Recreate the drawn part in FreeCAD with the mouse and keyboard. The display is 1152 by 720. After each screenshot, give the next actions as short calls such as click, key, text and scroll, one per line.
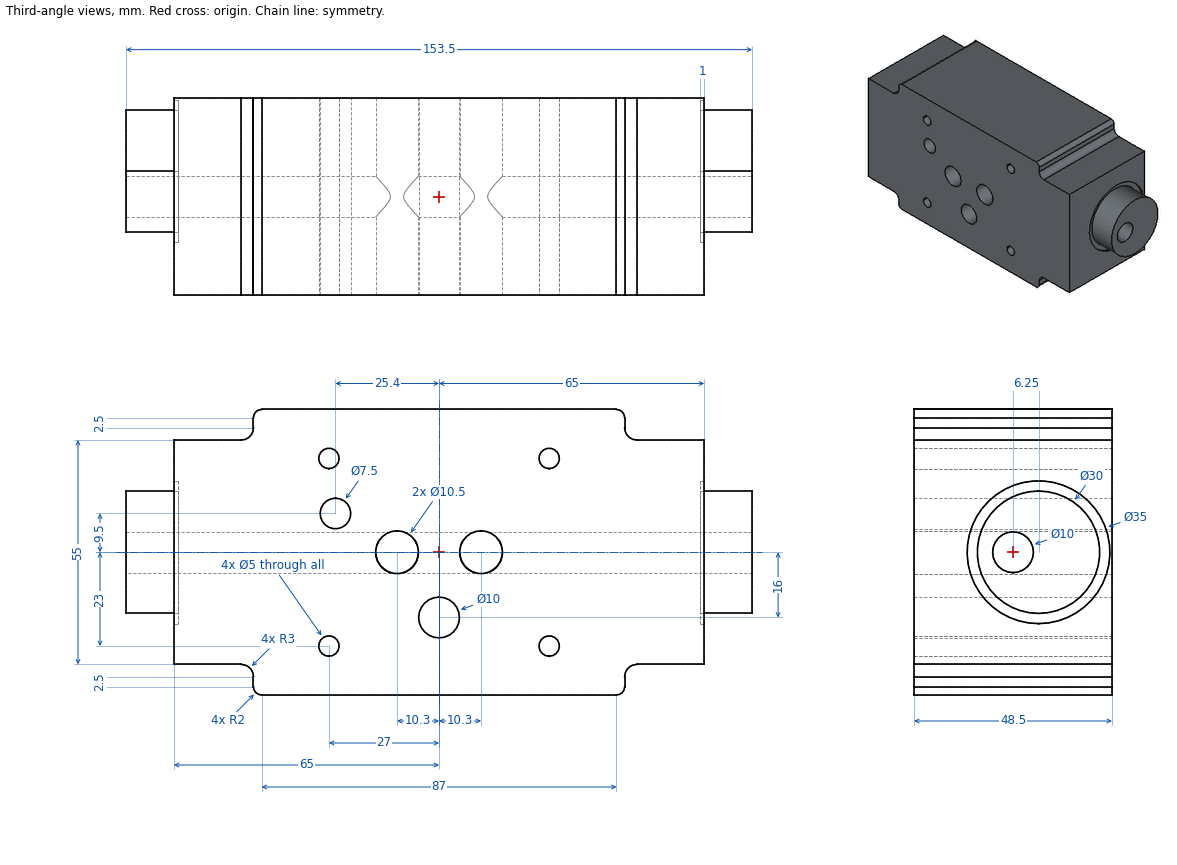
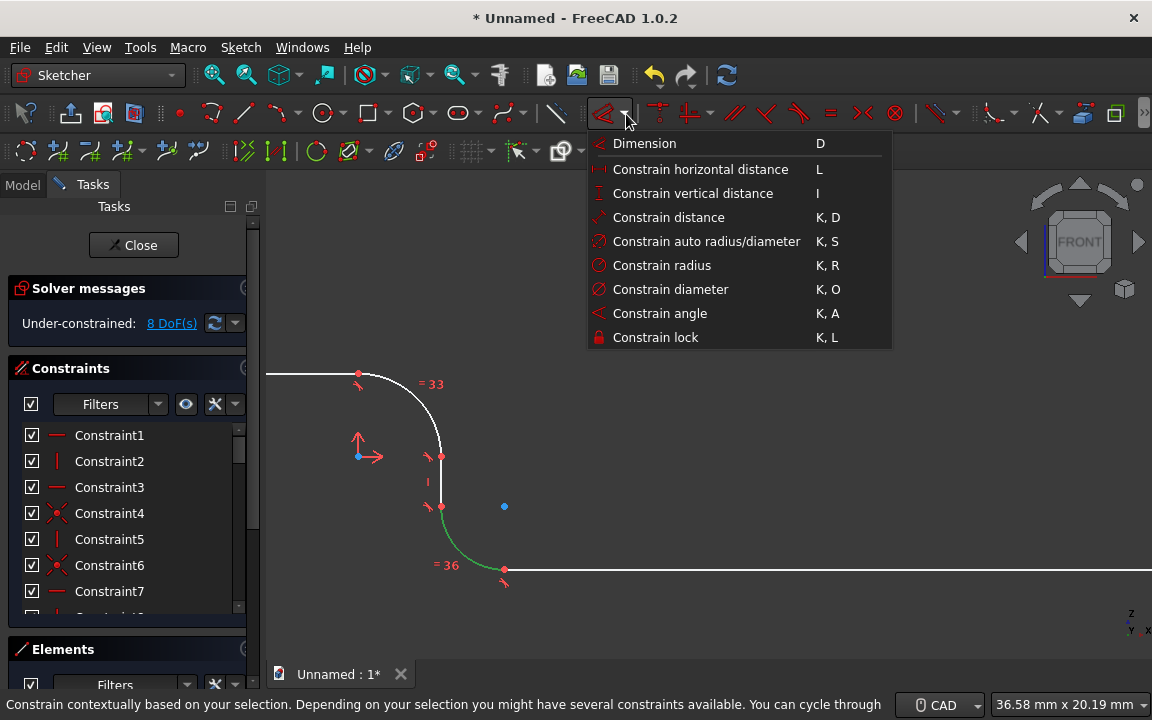
click(740, 265)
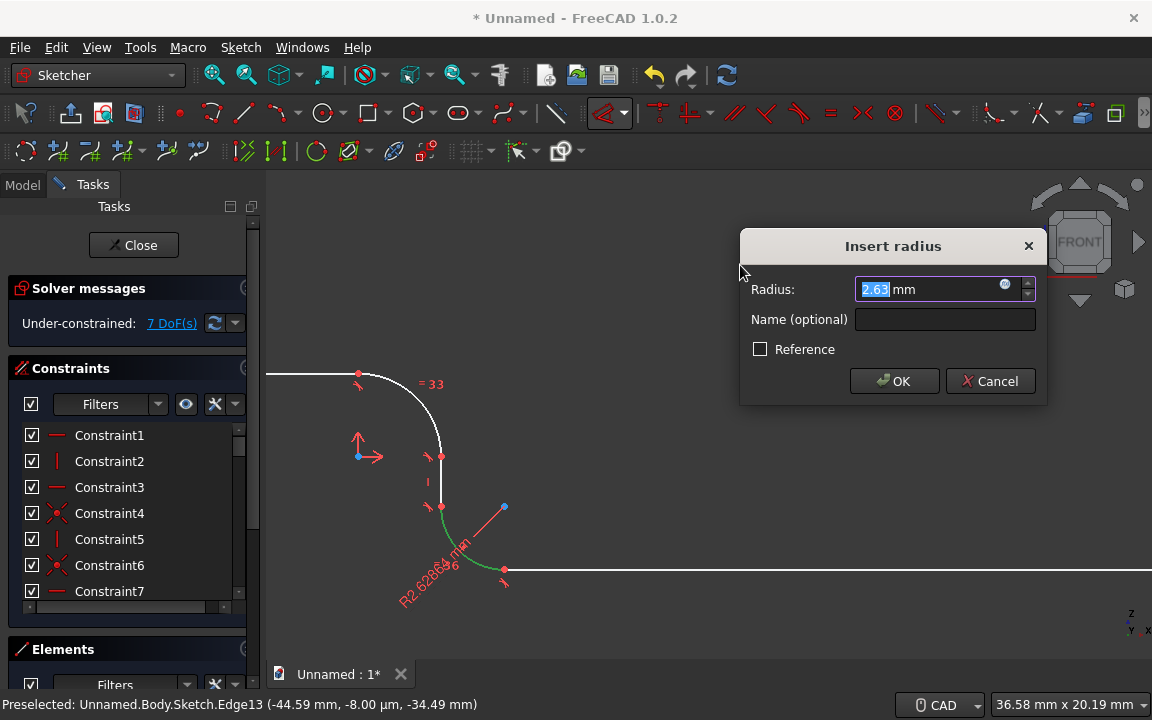
text(2)
key(Return)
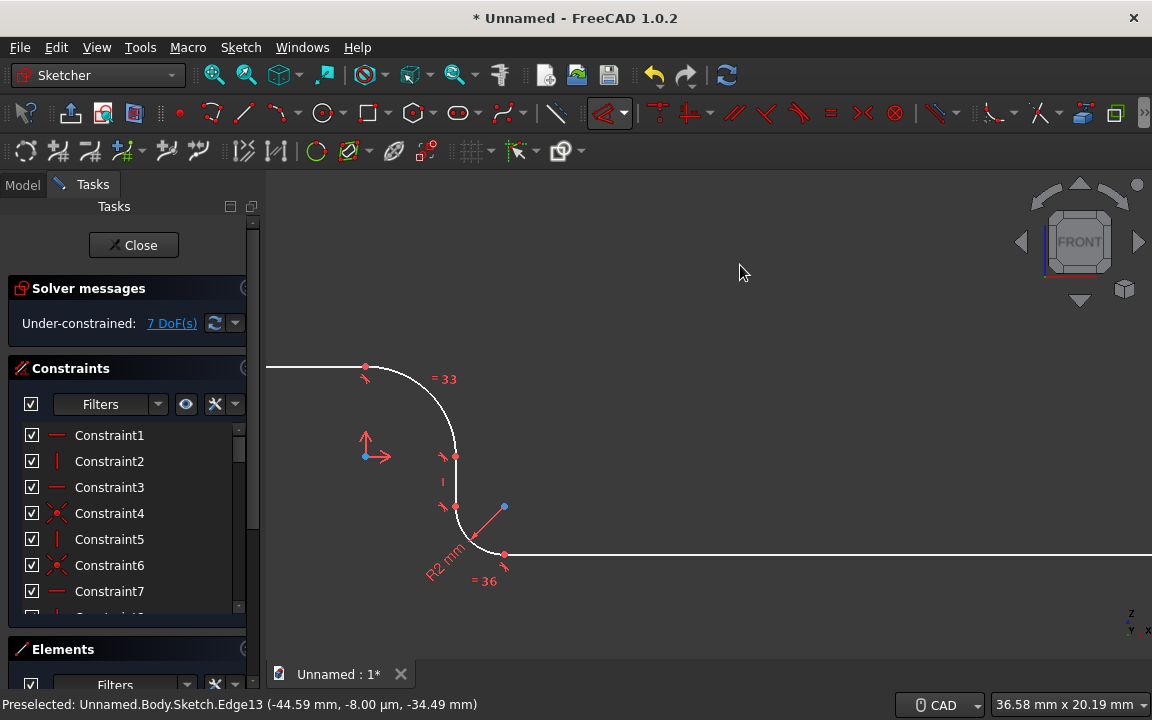
click(446, 416)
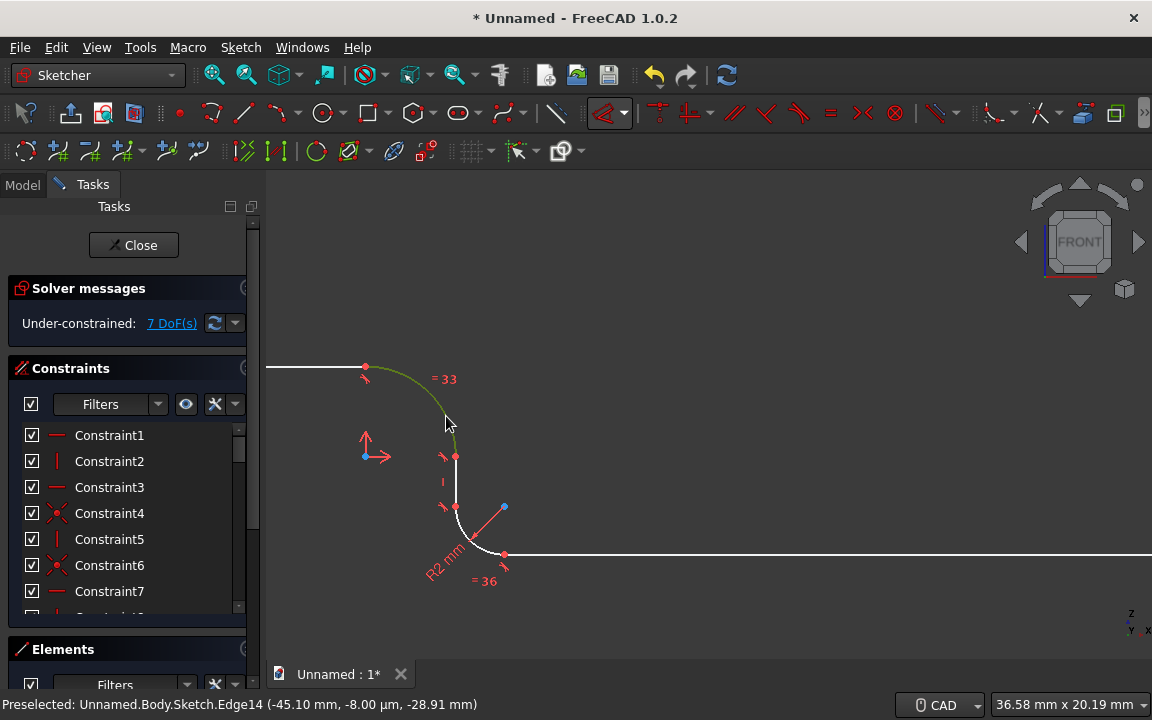
key(k)
key(r)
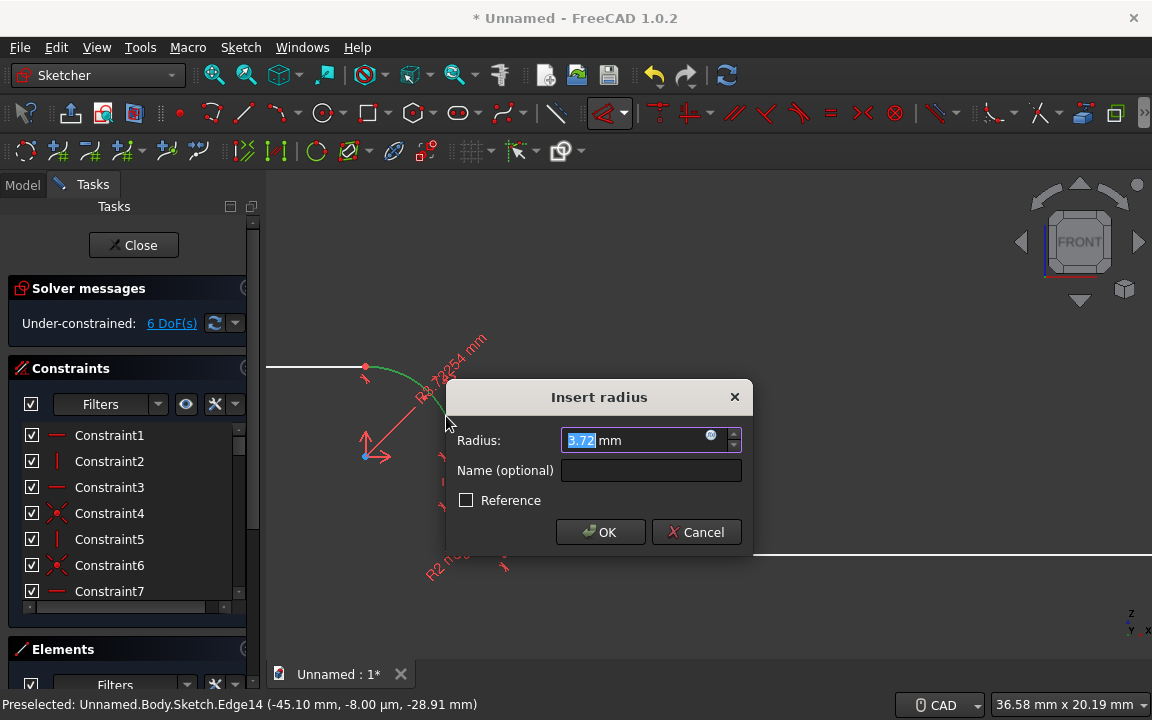
text(3)
key(Return)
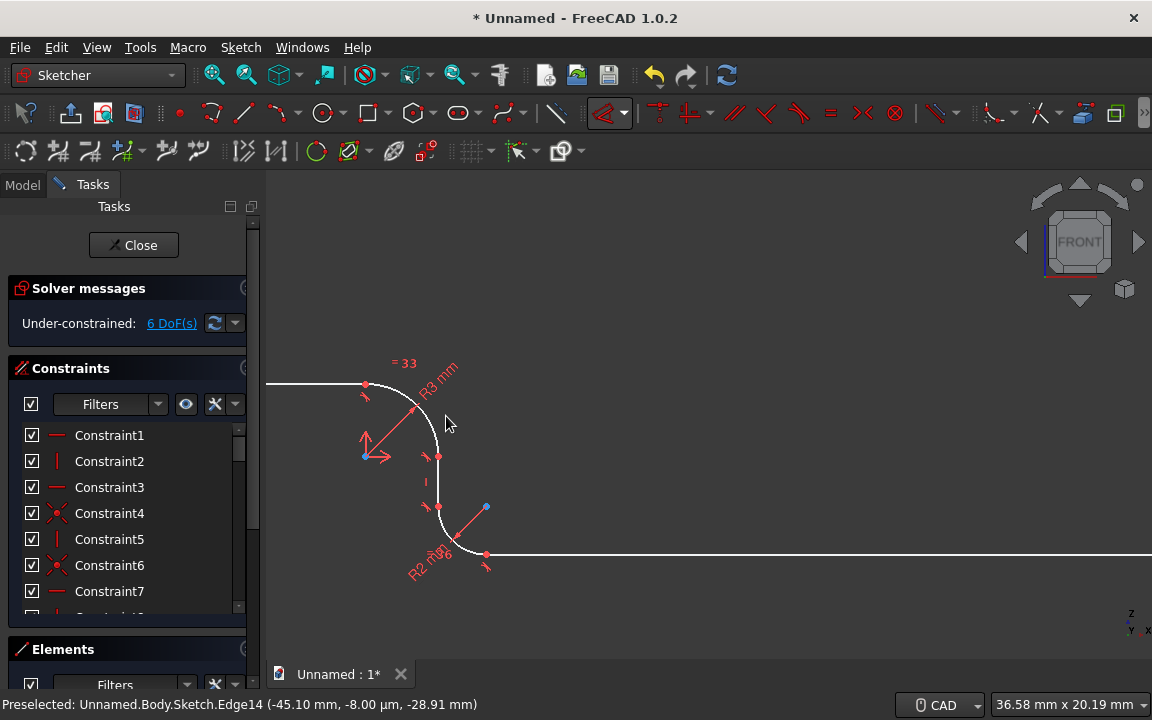
scroll(463, 553, down, 9)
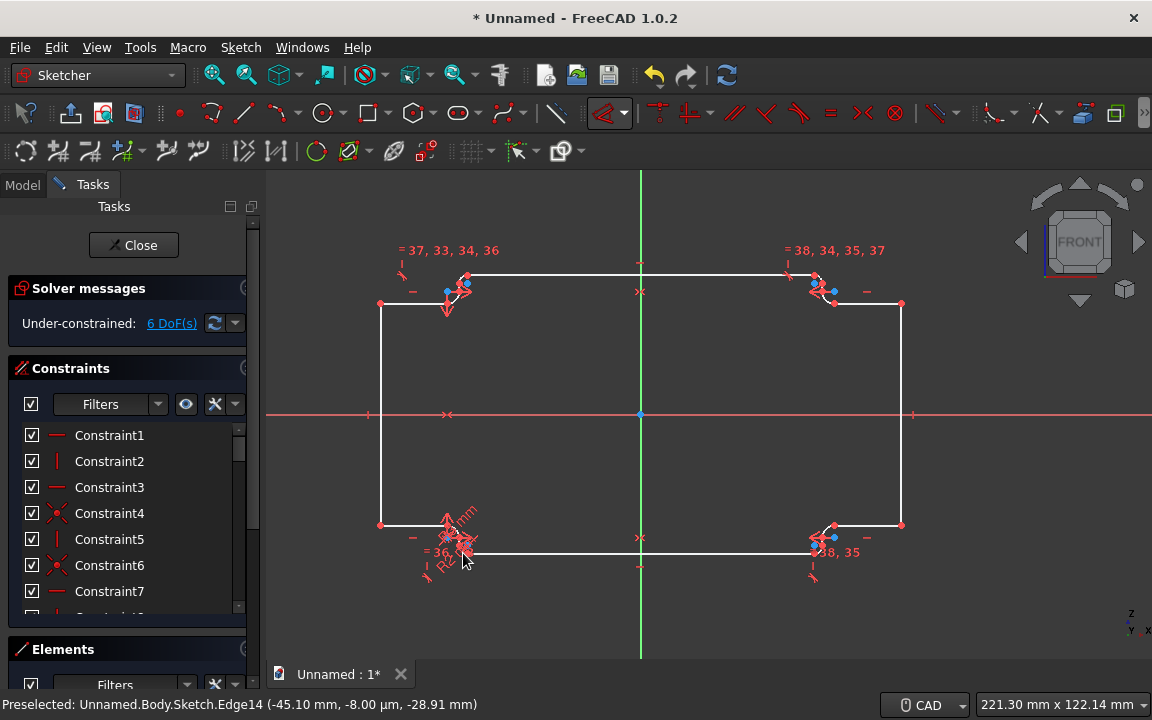
click(537, 554)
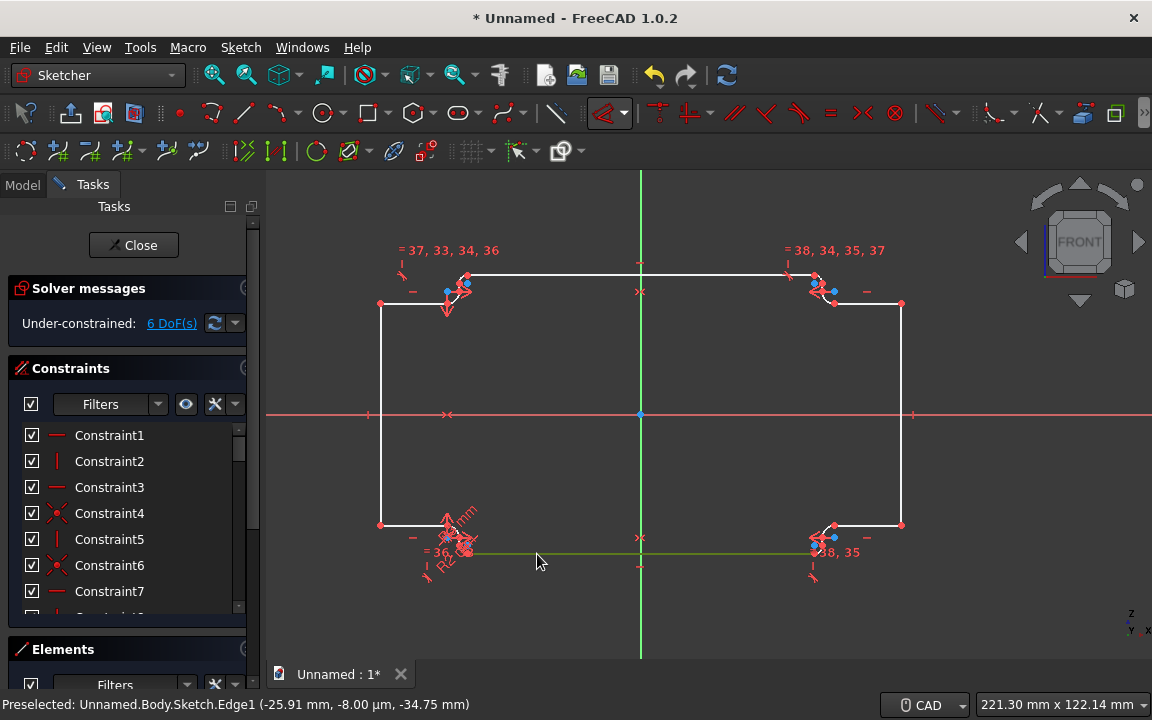
click(626, 114)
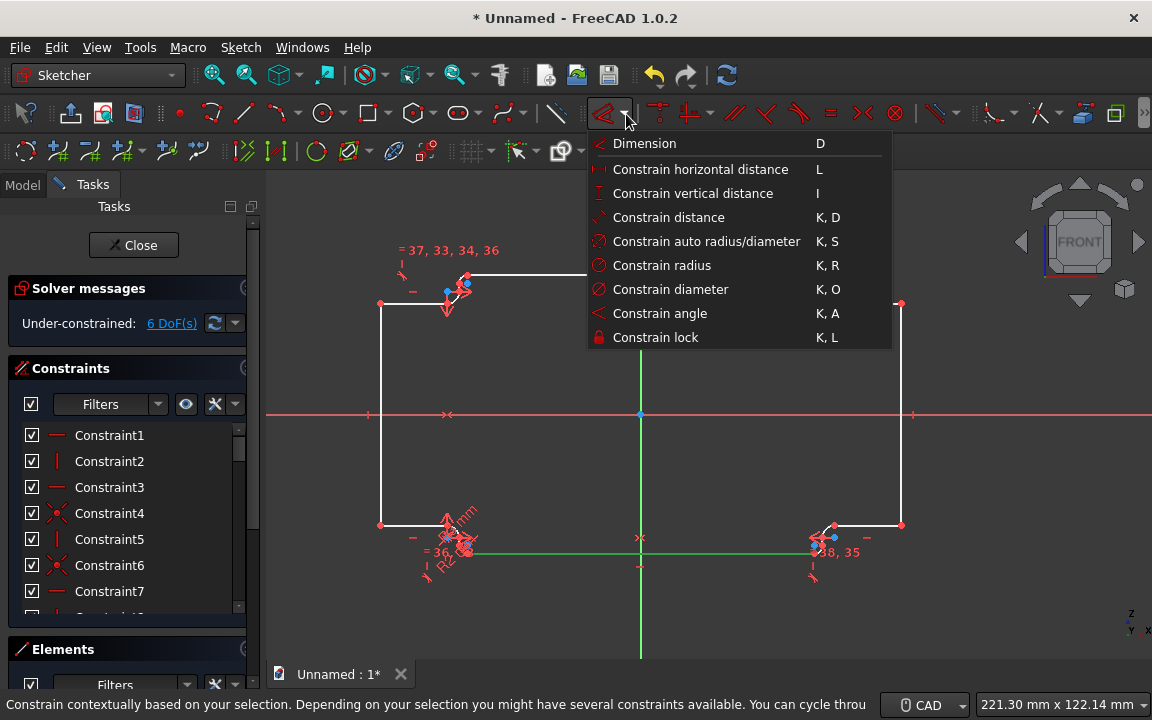
click(740, 169)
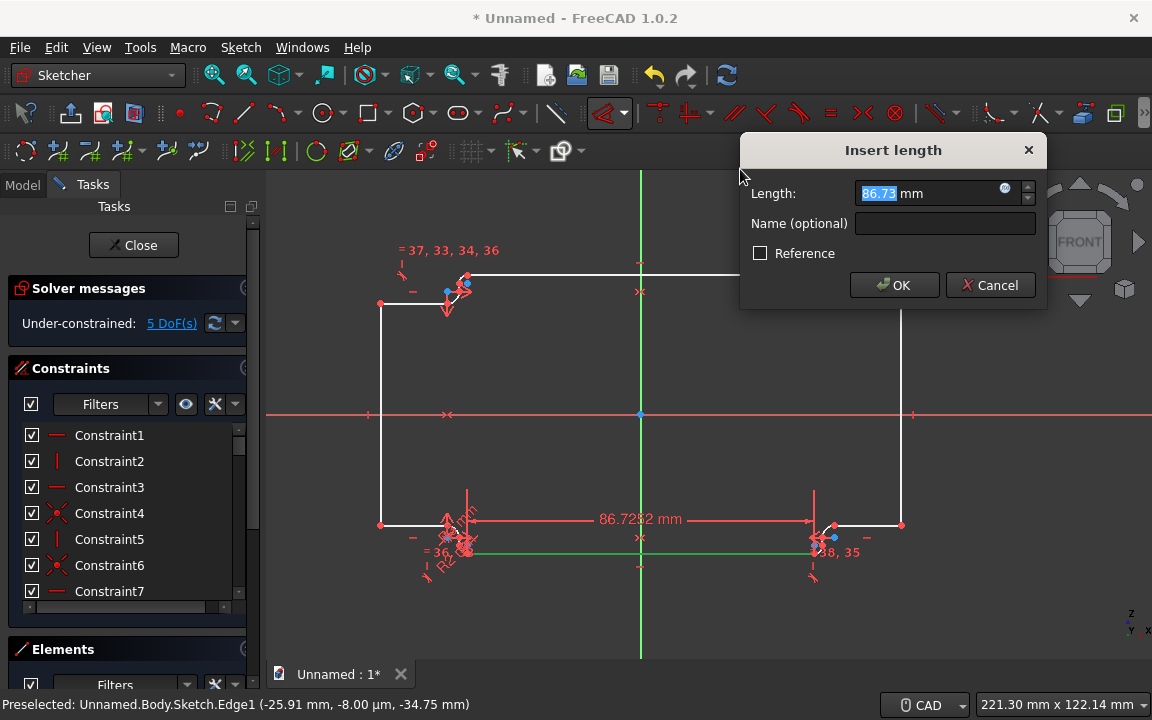
text(87)
key(Return)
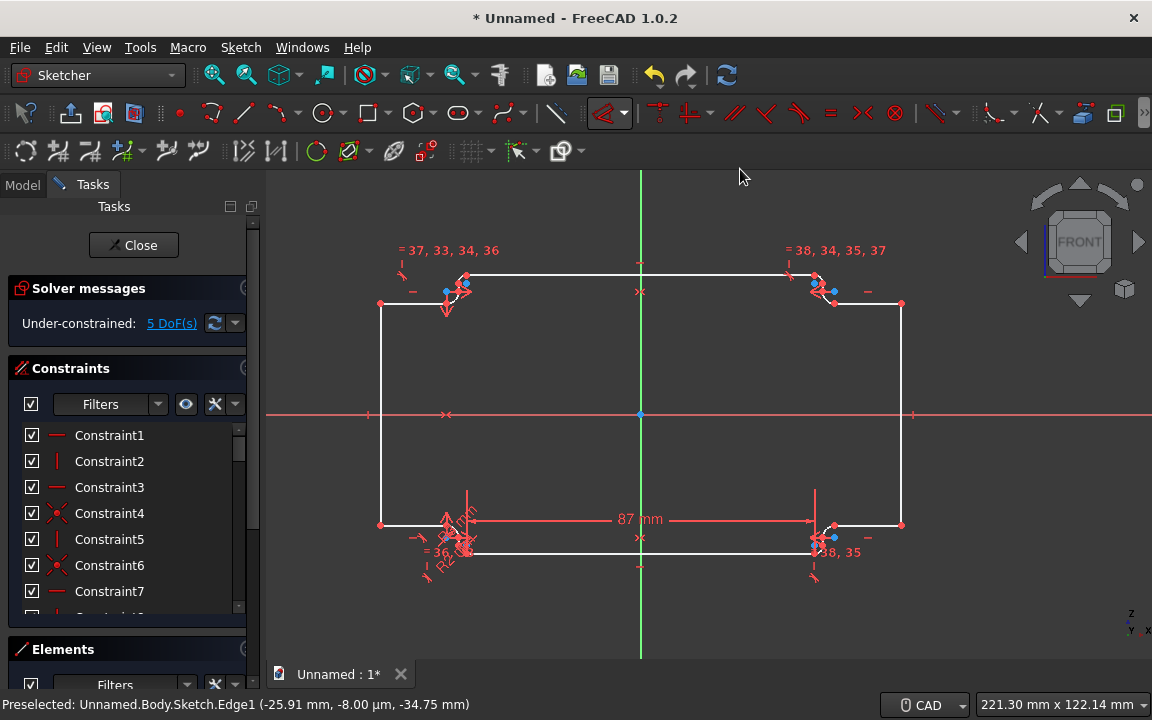
click(381, 459)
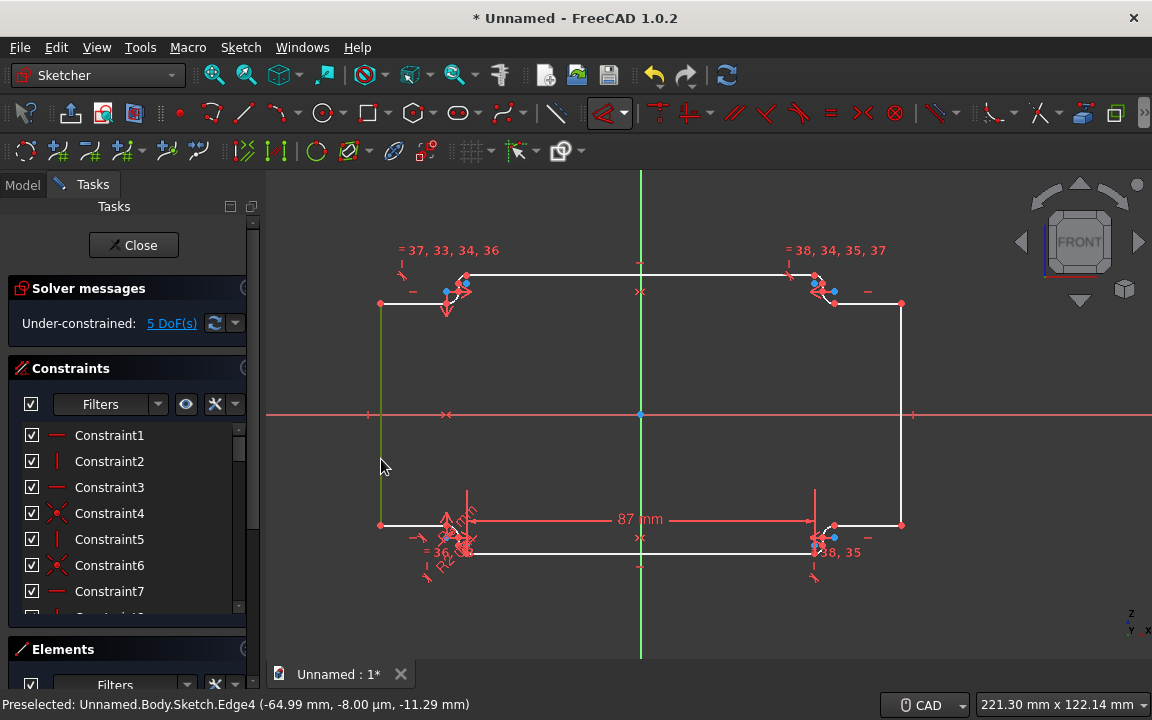
key(i)